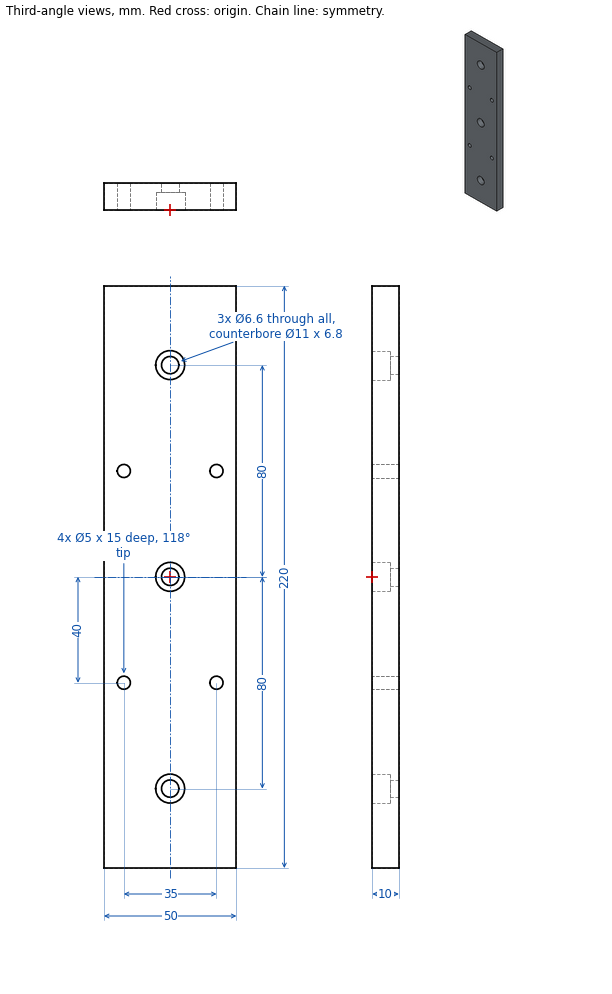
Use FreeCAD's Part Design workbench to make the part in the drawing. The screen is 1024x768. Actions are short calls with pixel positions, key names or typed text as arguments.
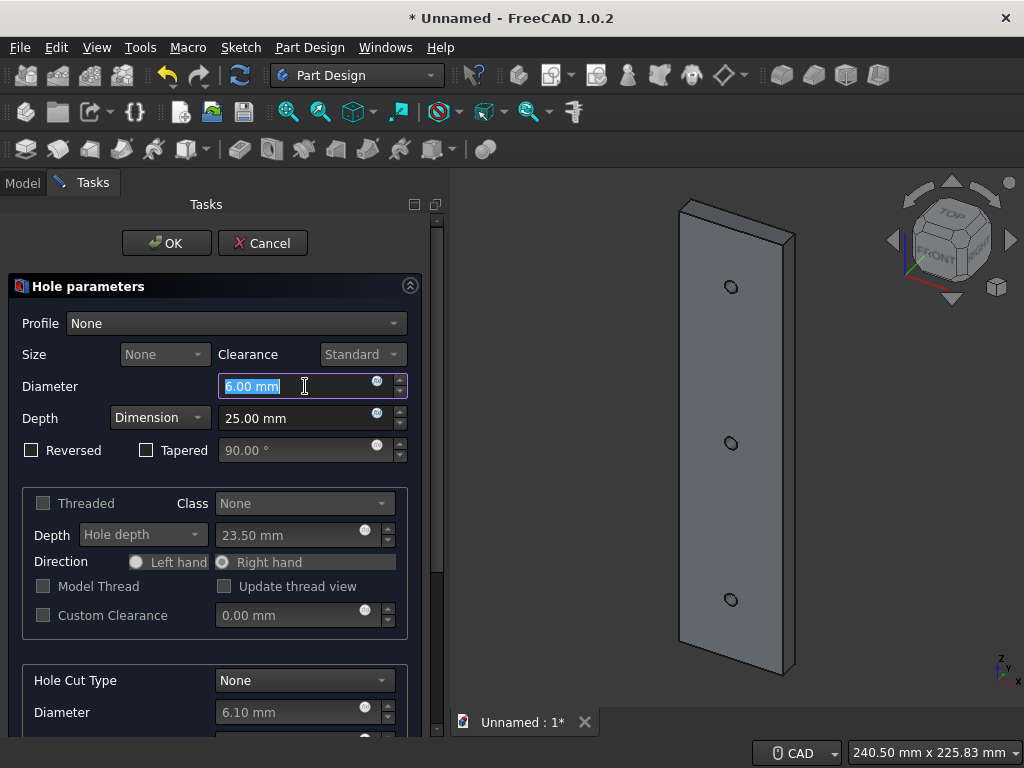
text(6.6)
key(Tab)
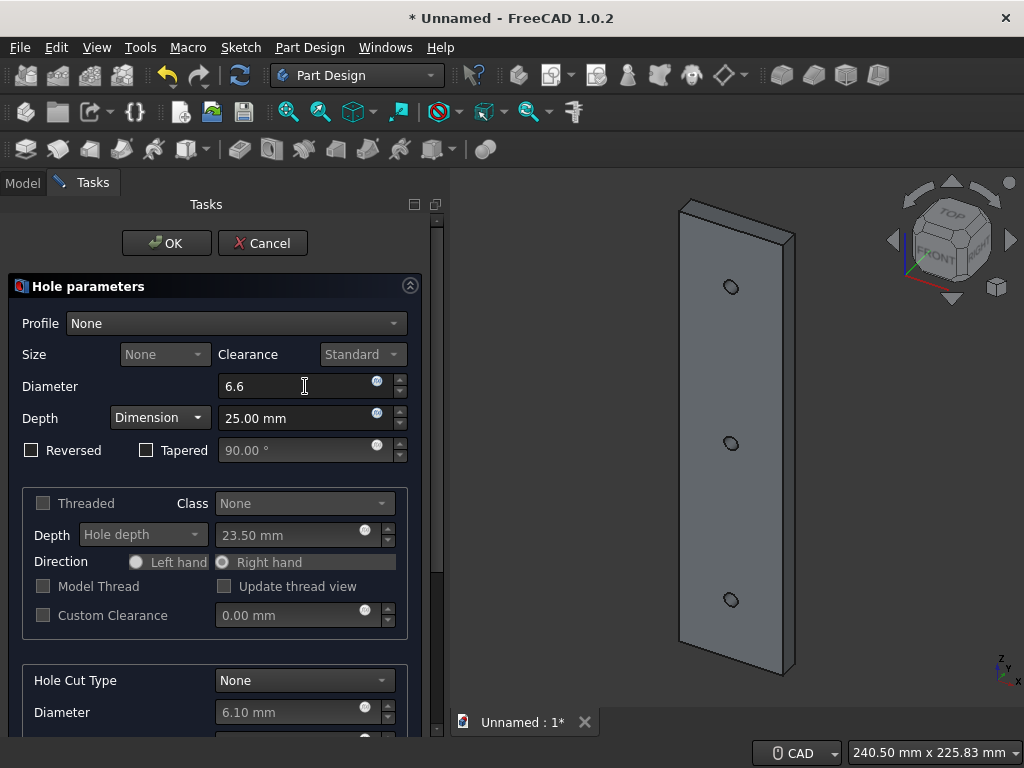
click(161, 418)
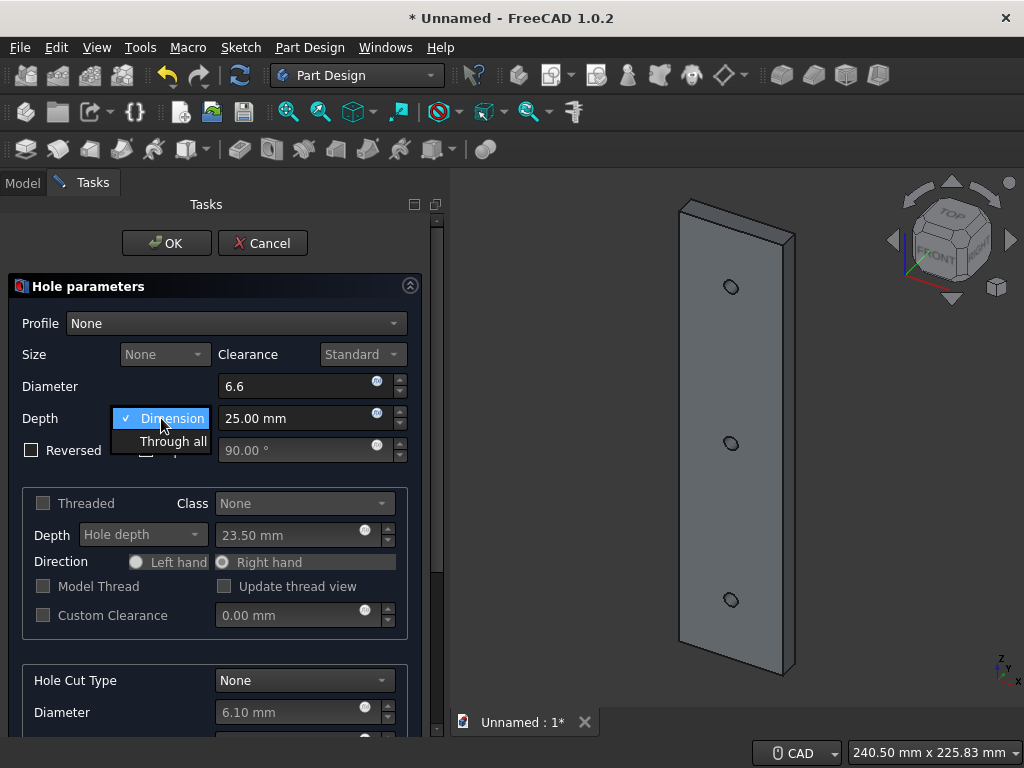
click(160, 442)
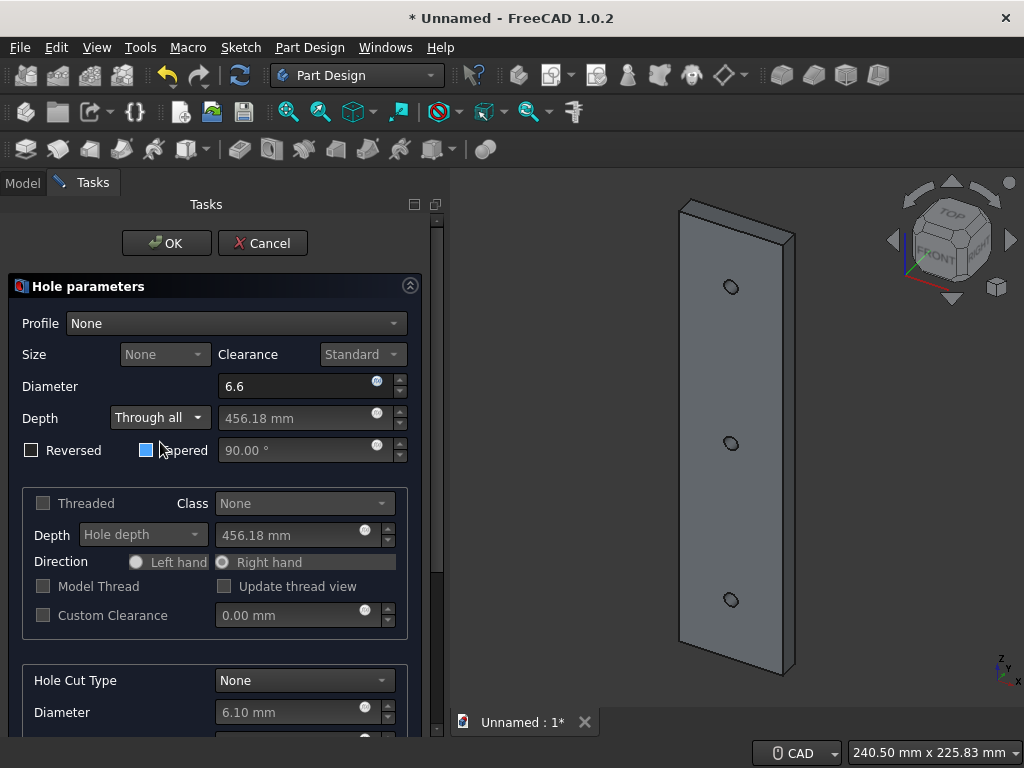
click(306, 680)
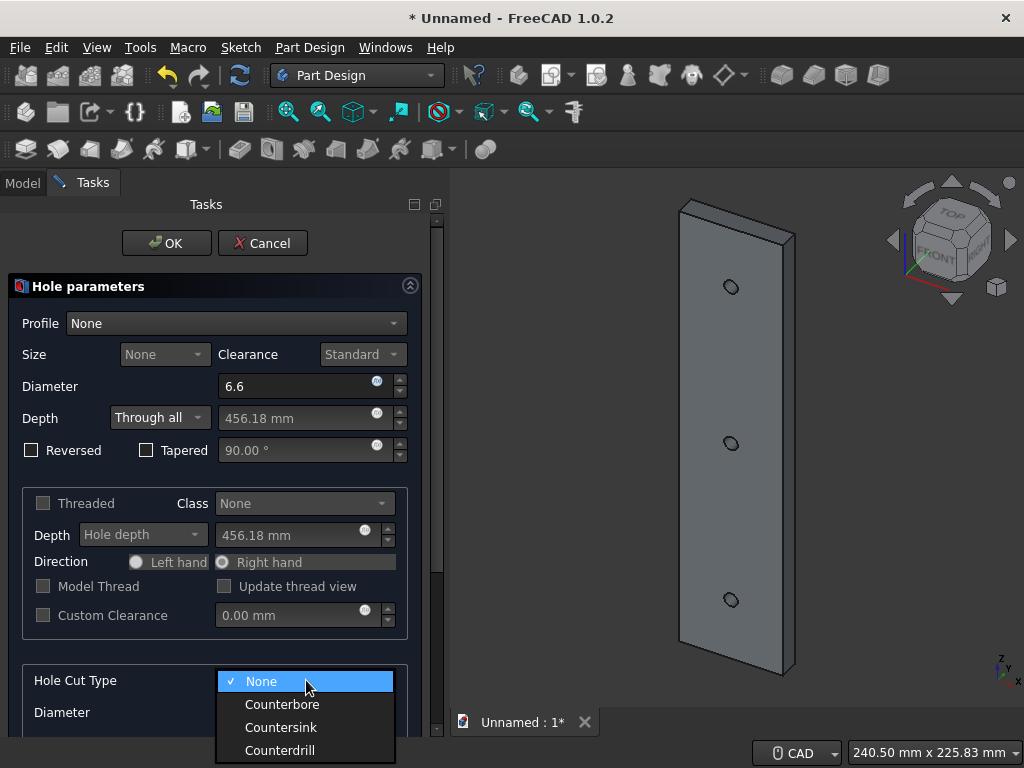
click(304, 704)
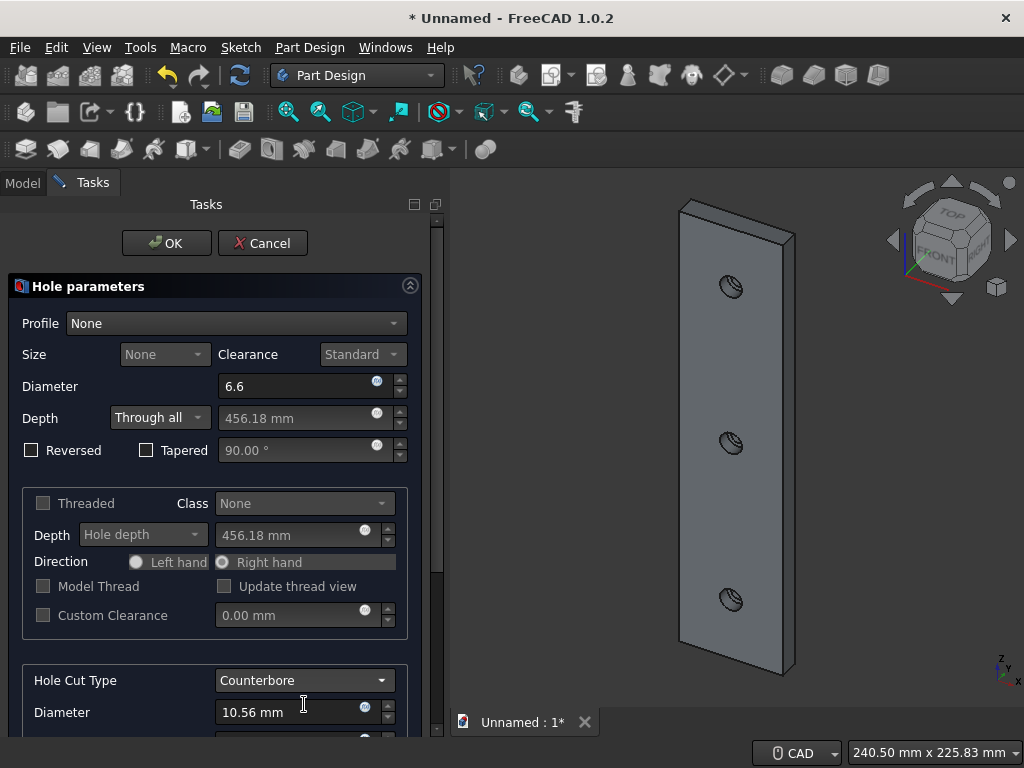
triple_click(298, 712)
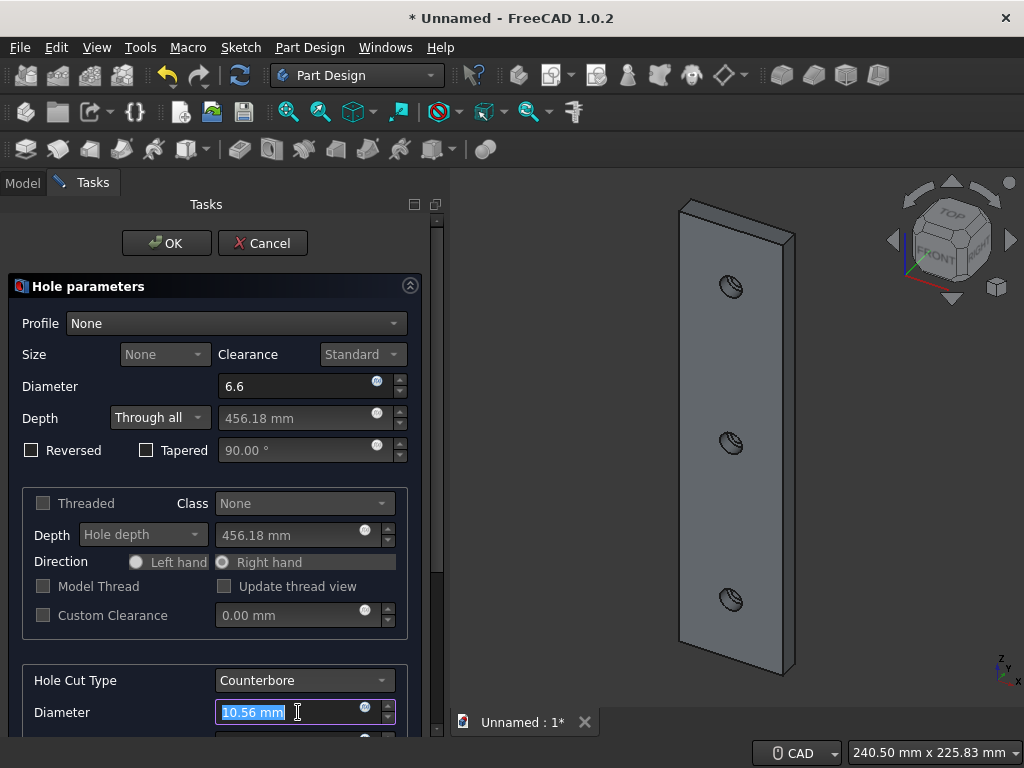
text(11)
key(Tab)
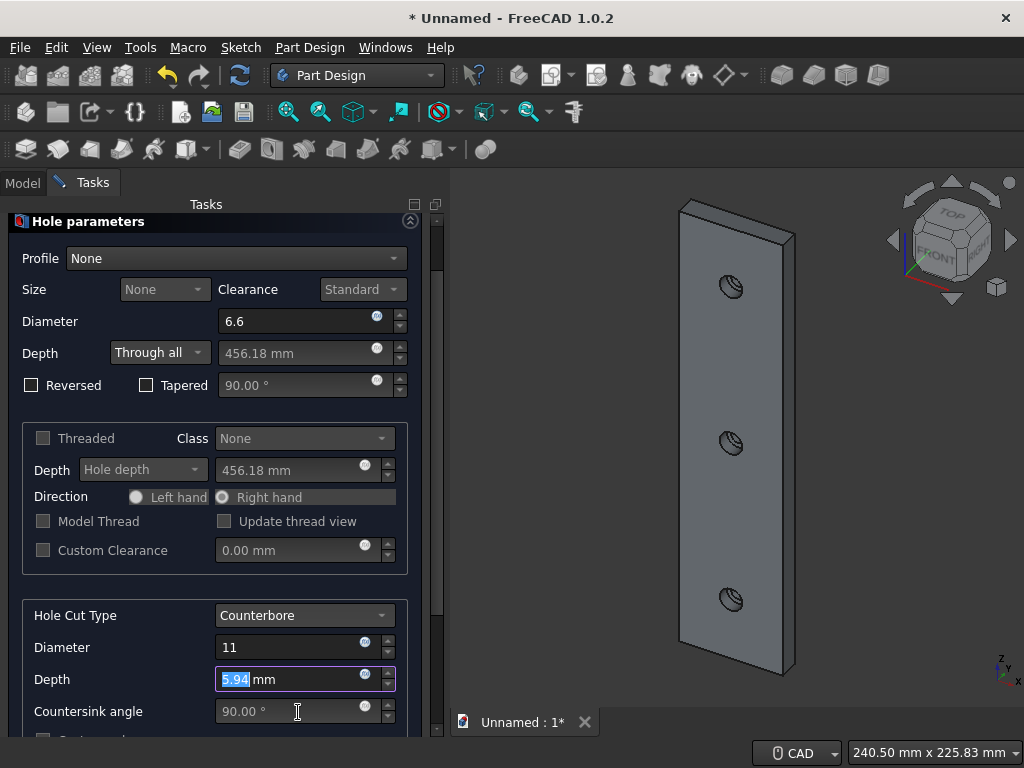
text(6.8)
key(Tab)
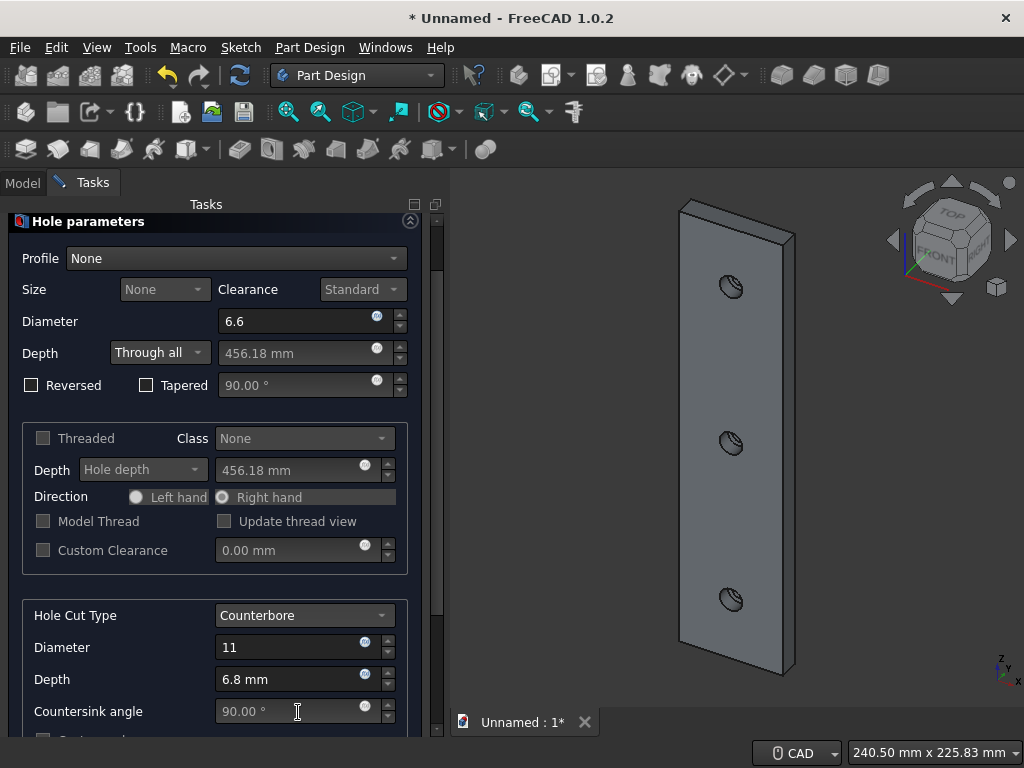
scroll(437, 475, up, 2)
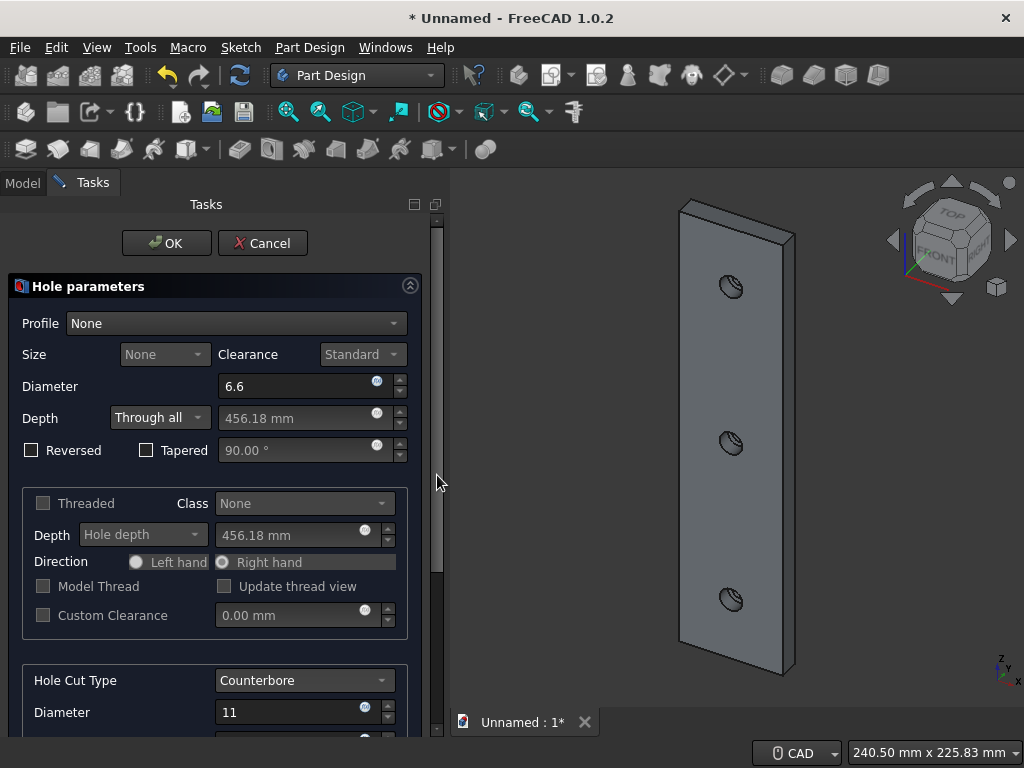
click(167, 243)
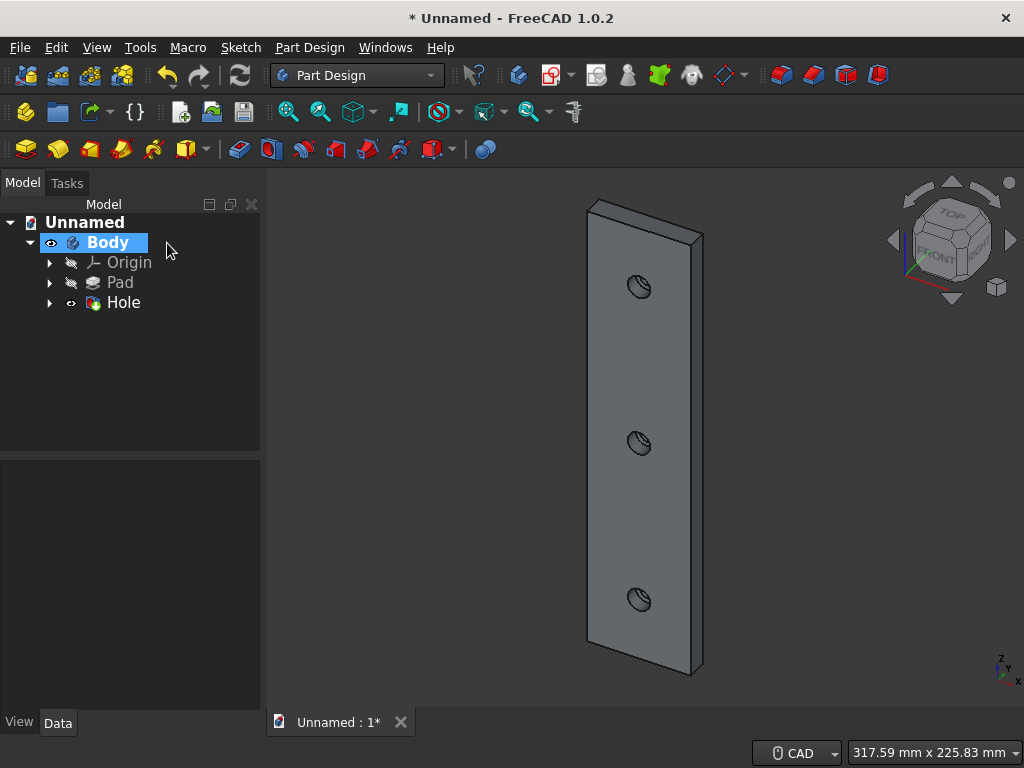
key(4)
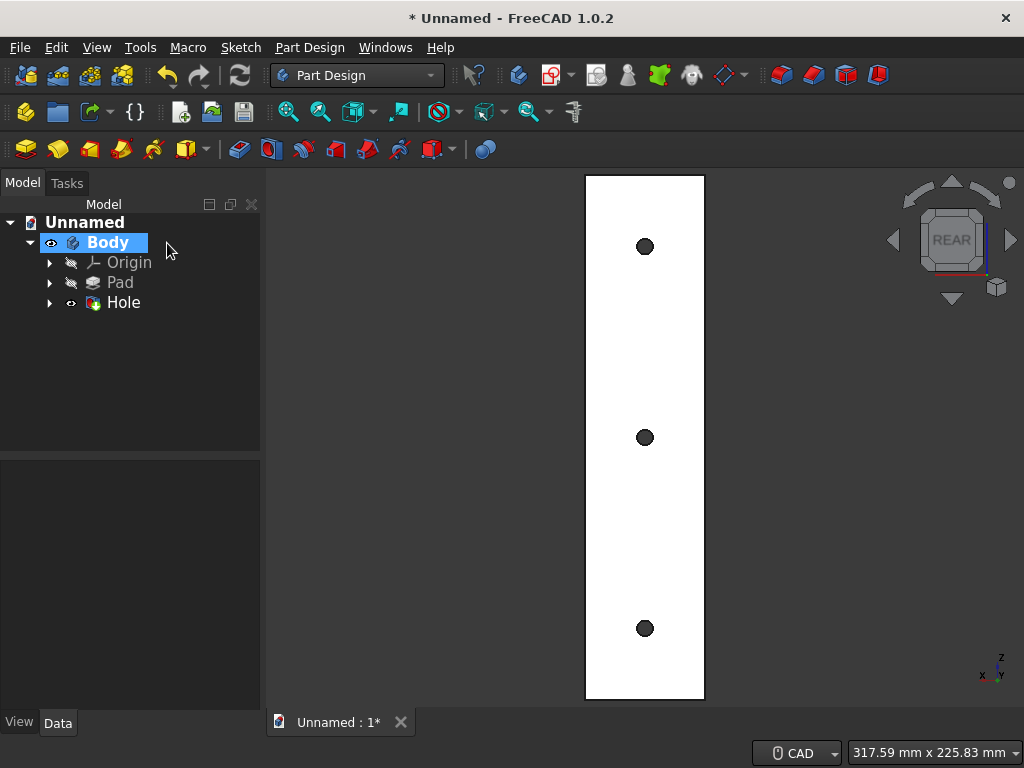
click(645, 361)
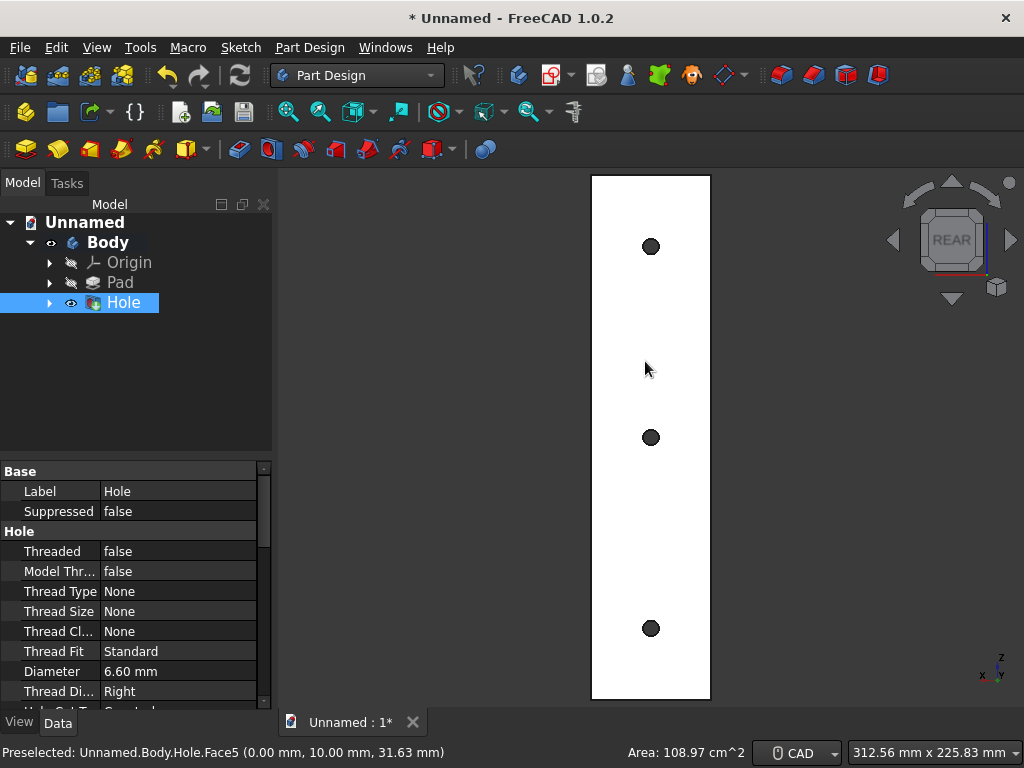
click(552, 76)